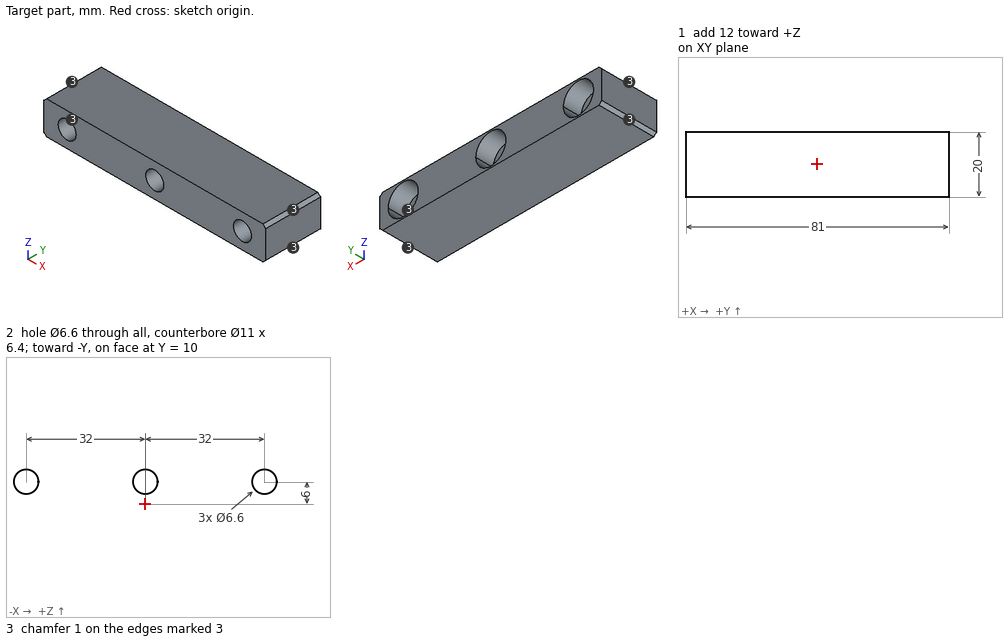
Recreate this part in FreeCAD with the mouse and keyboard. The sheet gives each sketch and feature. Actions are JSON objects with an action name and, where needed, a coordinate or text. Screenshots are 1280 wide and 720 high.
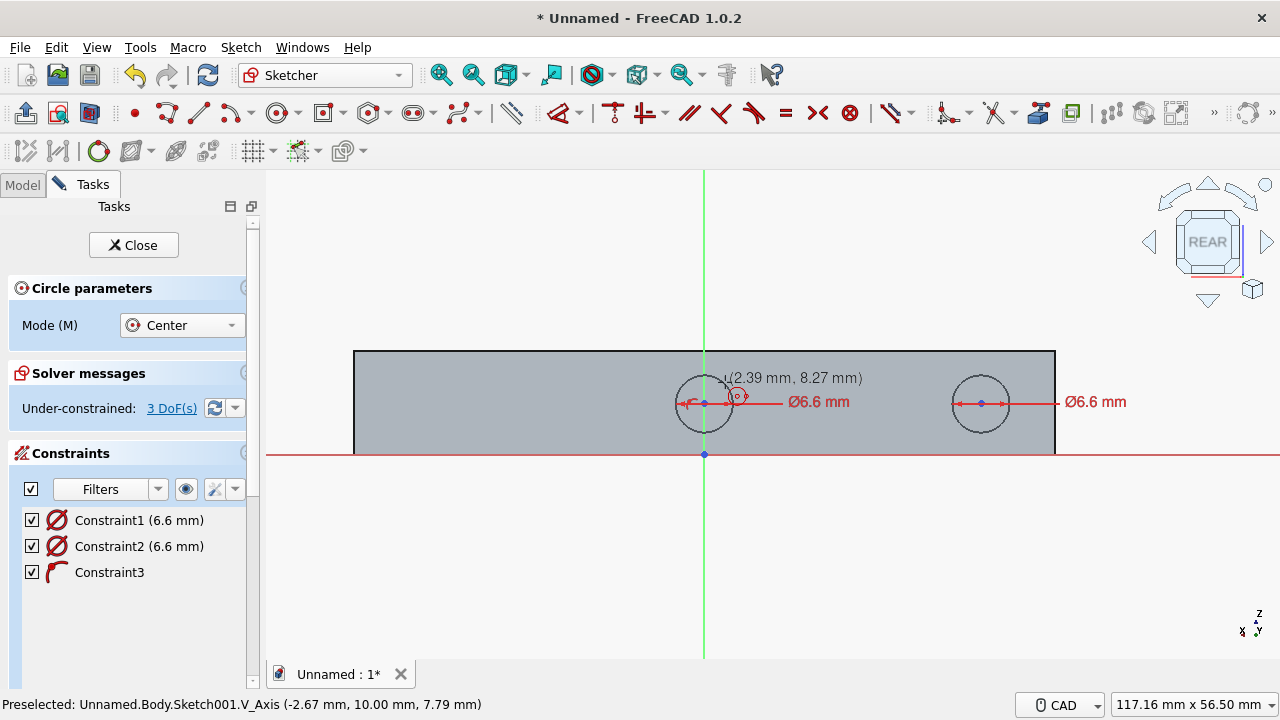
{"action": "left_click", "coordinate": [427, 403]}
{"action": "mouse_move", "coordinate": [448, 382]}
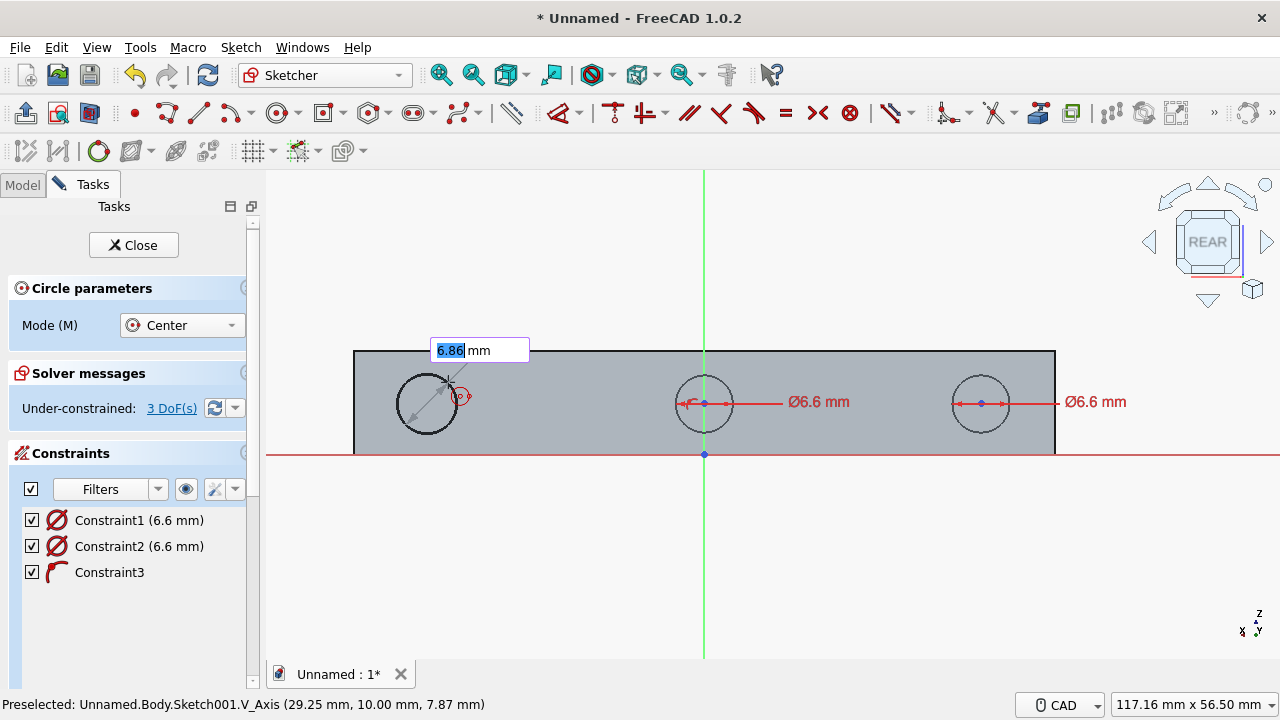
{"action": "type", "text": "6.6"}
{"action": "key", "text": "Return"}
{"action": "key", "text": "Escape"}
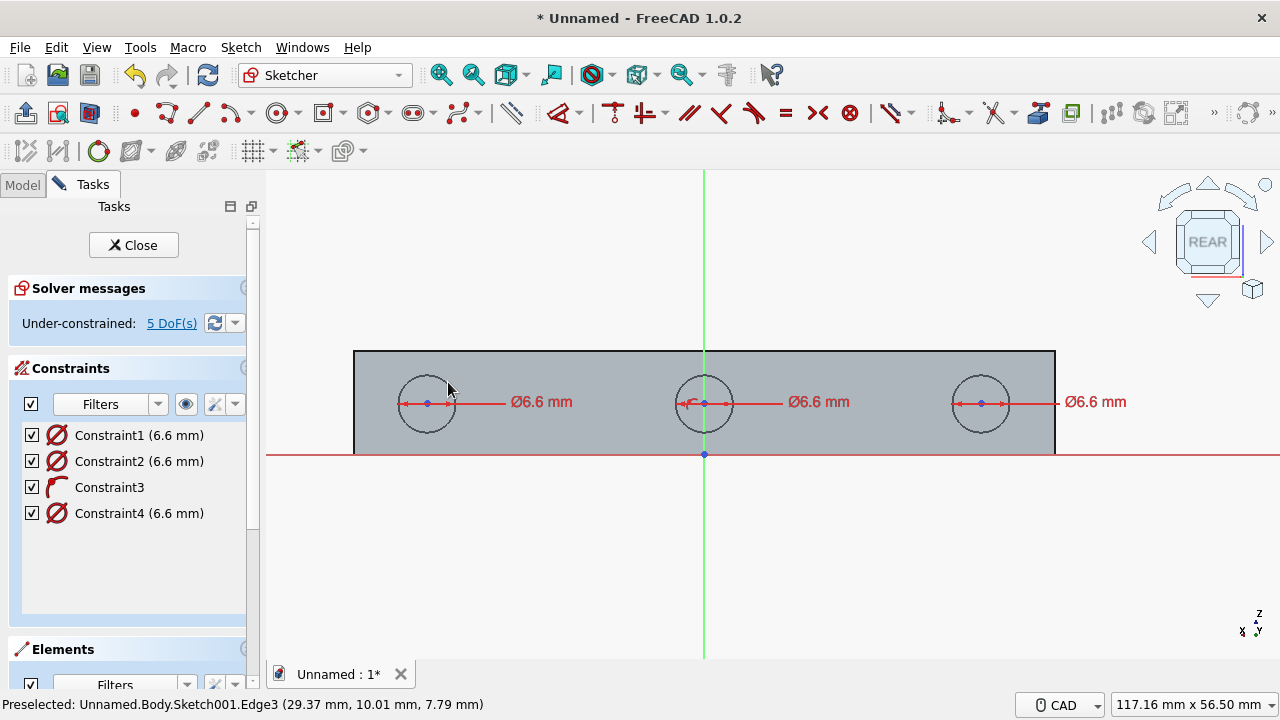
{"action": "left_click", "coordinate": [981, 404]}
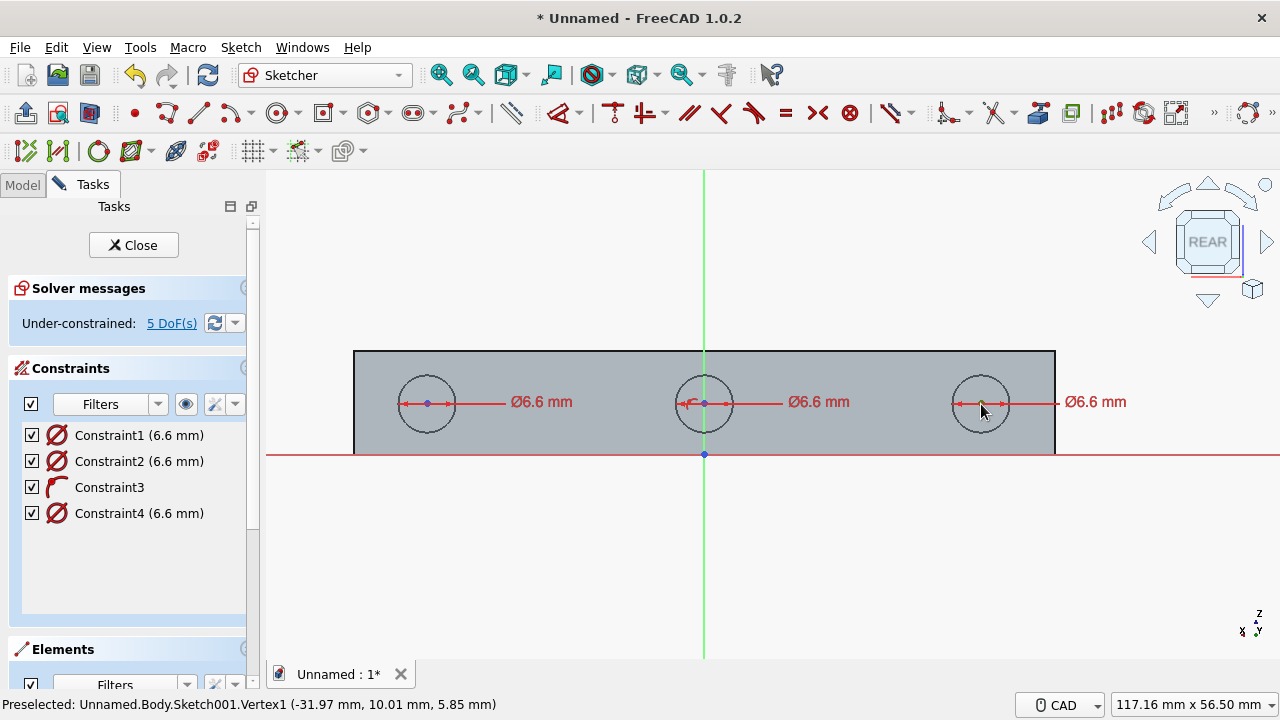
{"action": "left_click", "coordinate": [704, 404]}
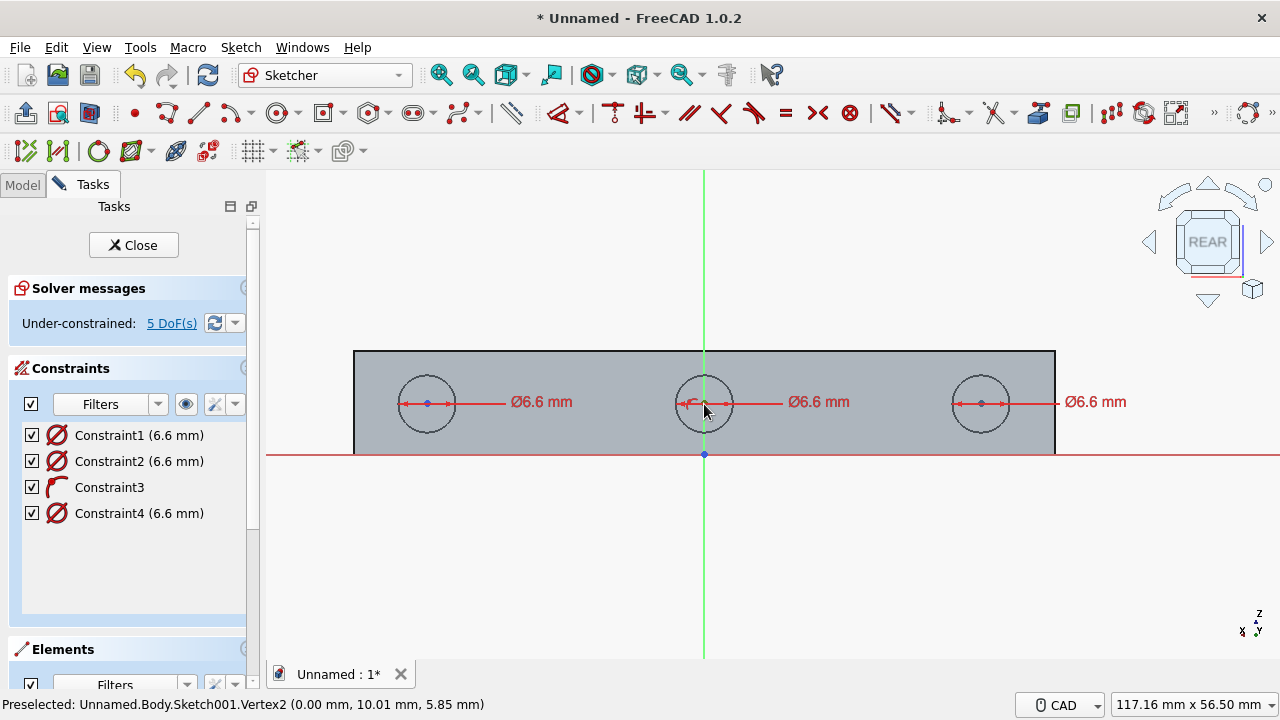
{"action": "left_click", "coordinate": [668, 114]}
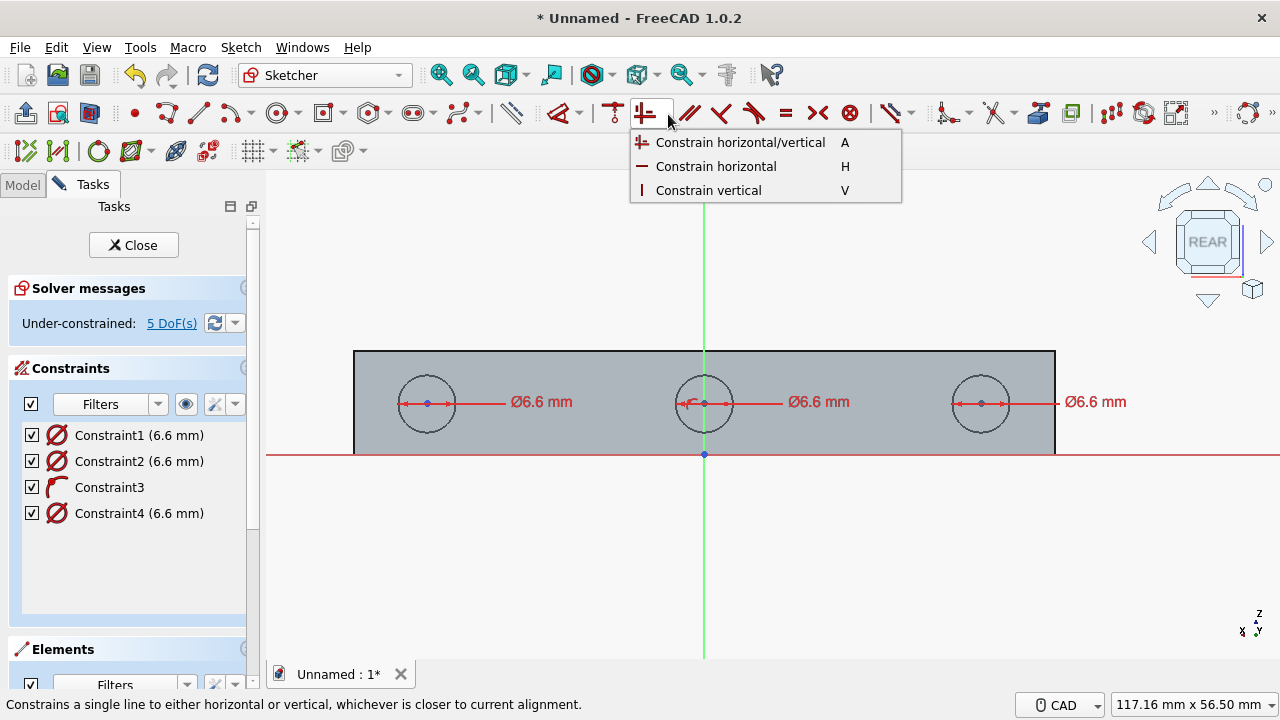
{"action": "left_click", "coordinate": [766, 166]}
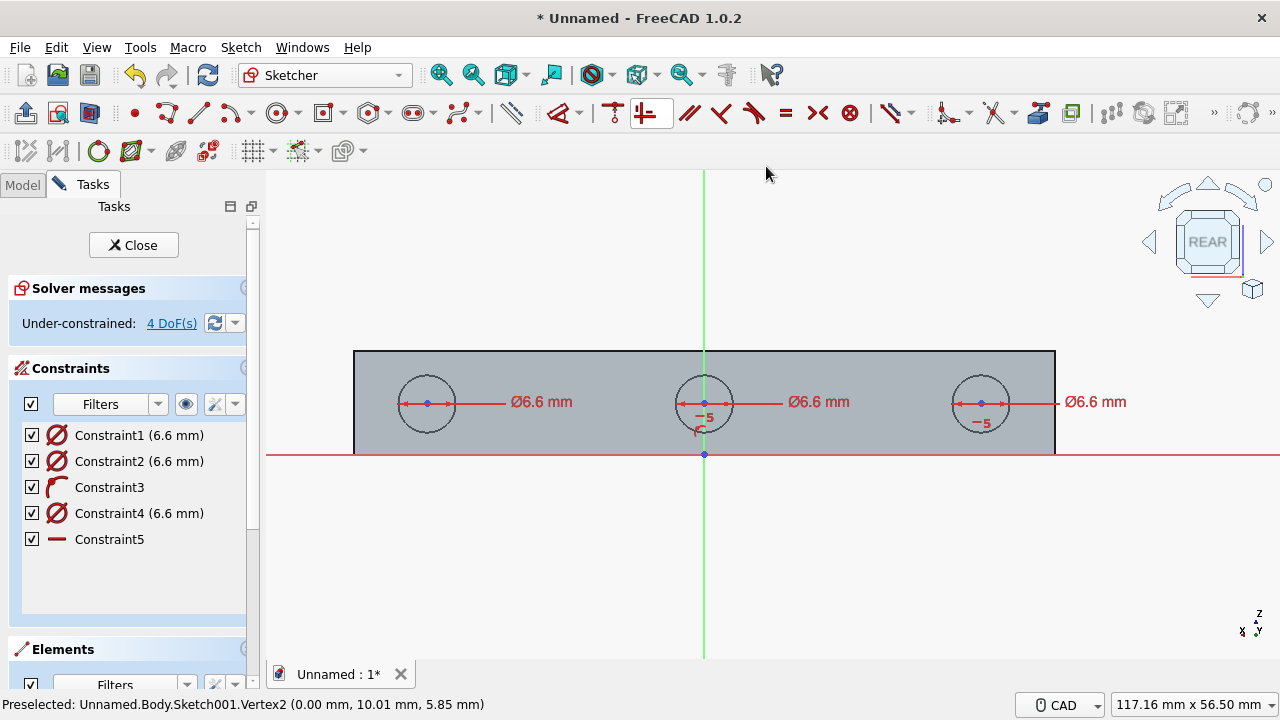
{"action": "left_click", "coordinate": [704, 404]}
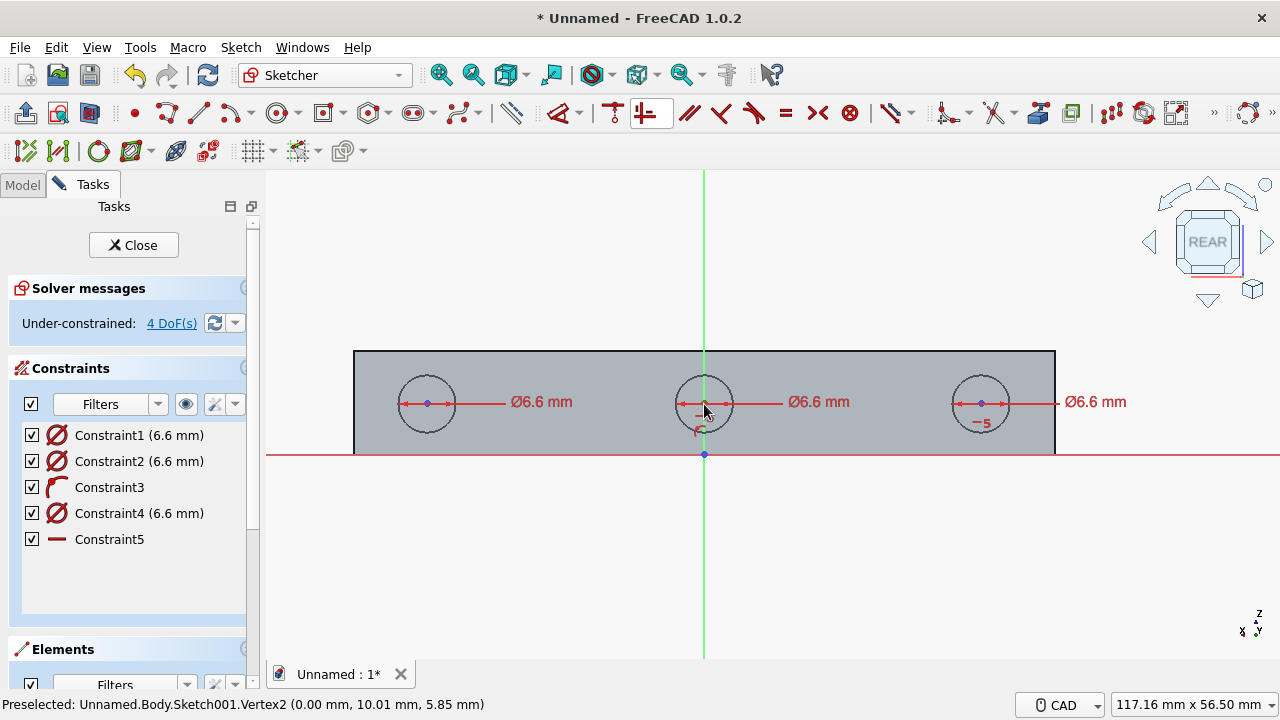
{"action": "left_click", "coordinate": [427, 404]}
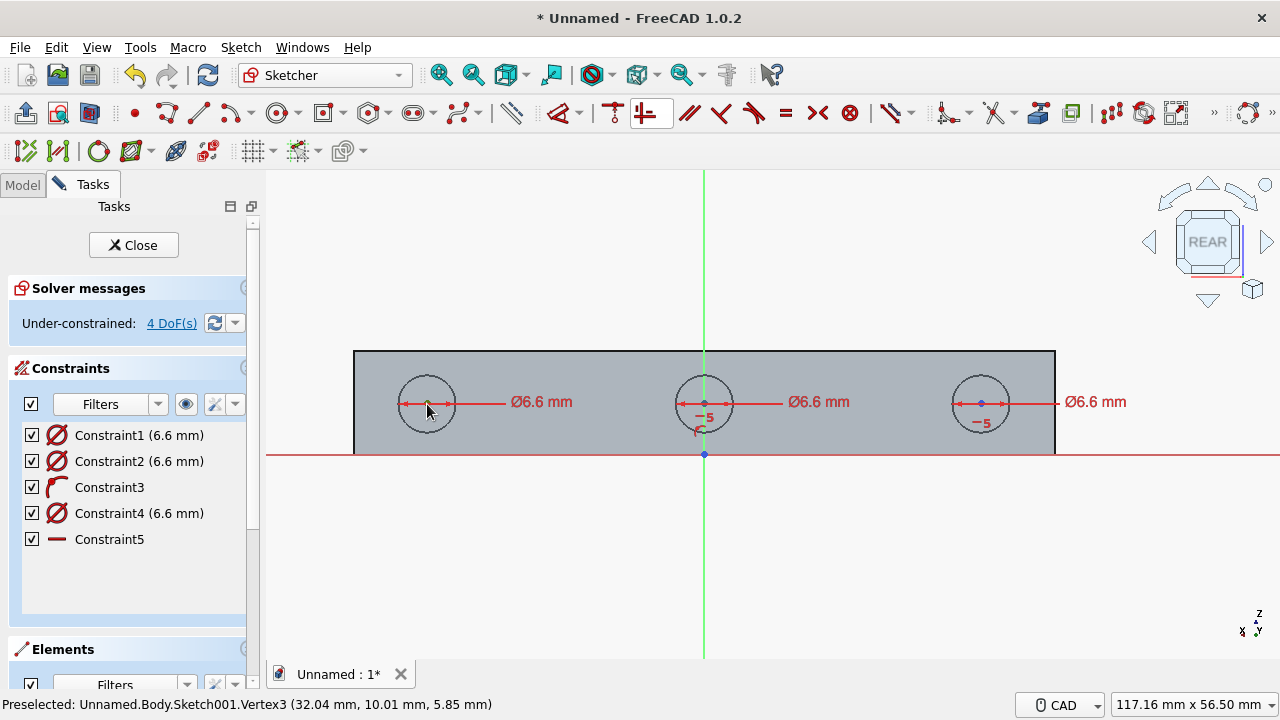
{"action": "key", "text": "h"}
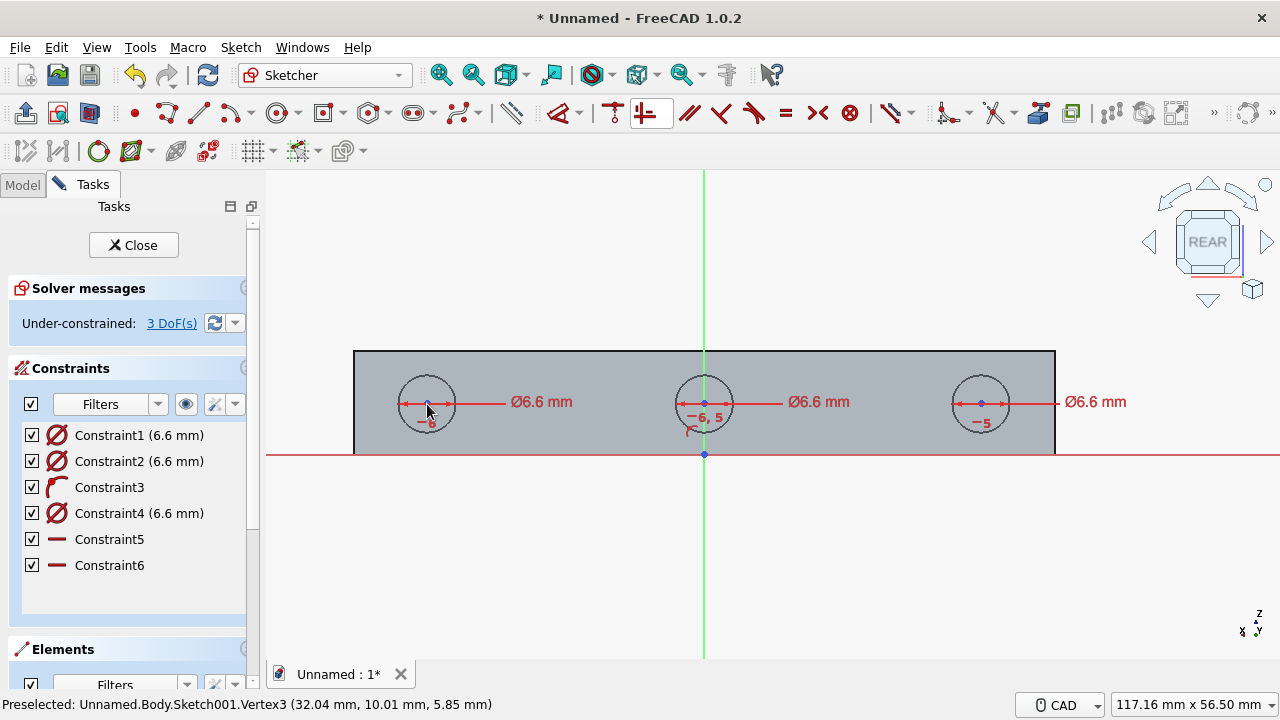
{"action": "left_click", "coordinate": [558, 114]}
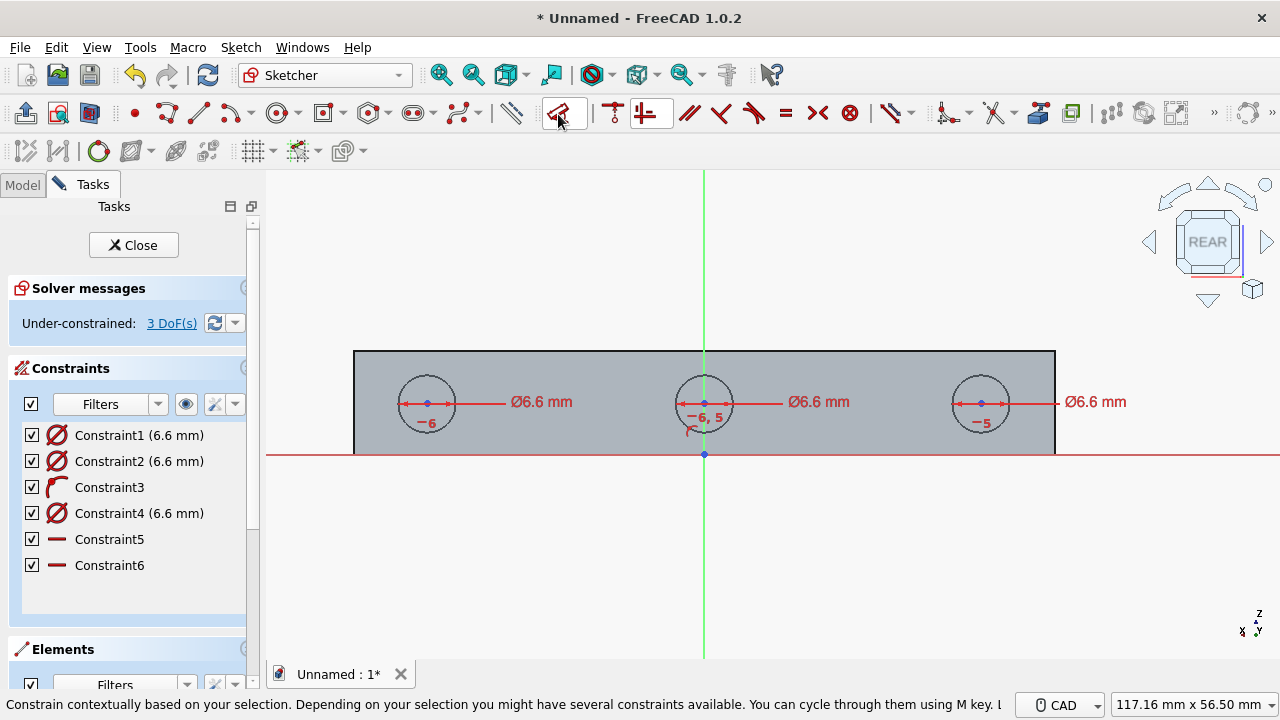
{"action": "left_click", "coordinate": [981, 404]}
{"action": "left_click", "coordinate": [1015, 429]}